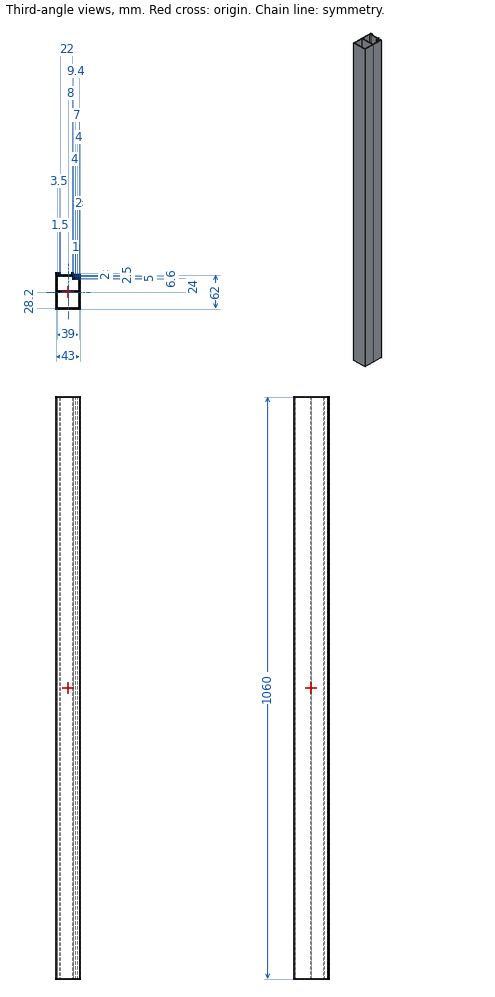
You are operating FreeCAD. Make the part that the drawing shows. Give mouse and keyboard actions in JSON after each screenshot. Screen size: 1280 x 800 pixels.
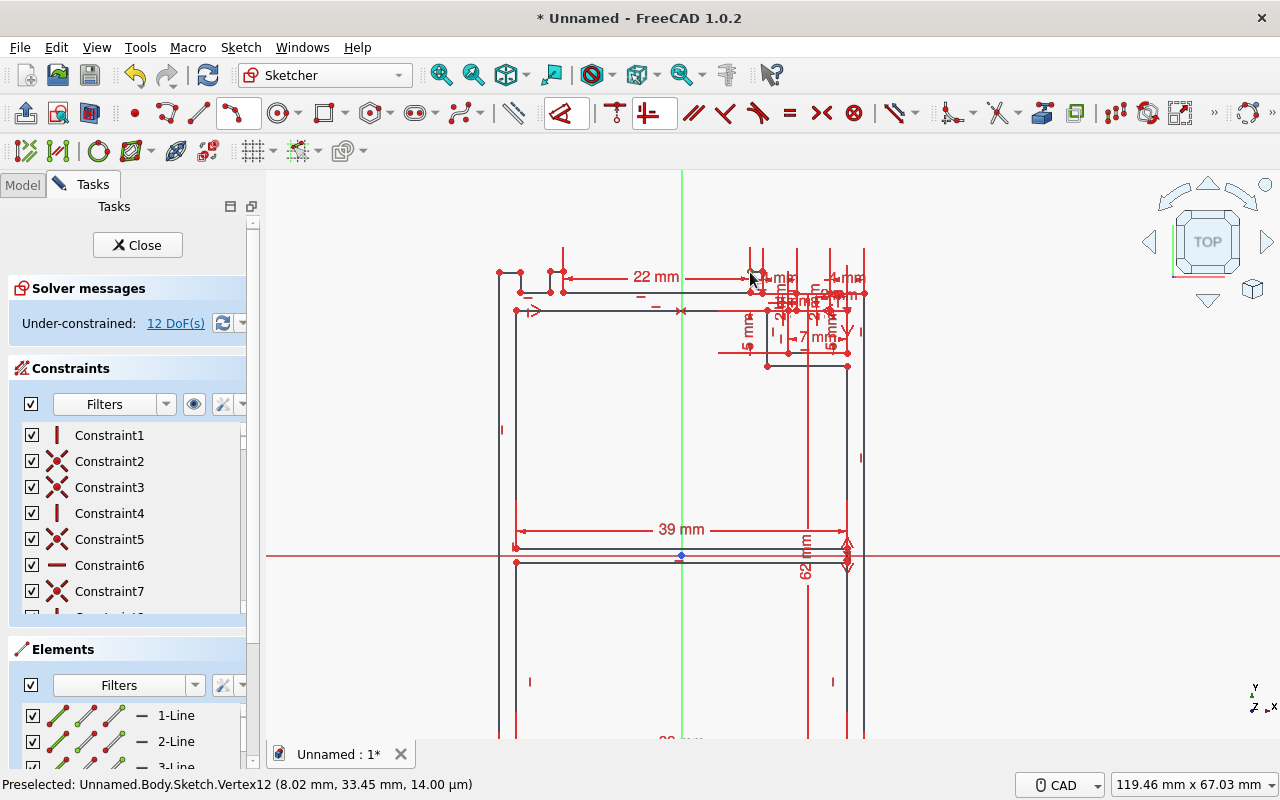
{"action": "key", "text": "l"}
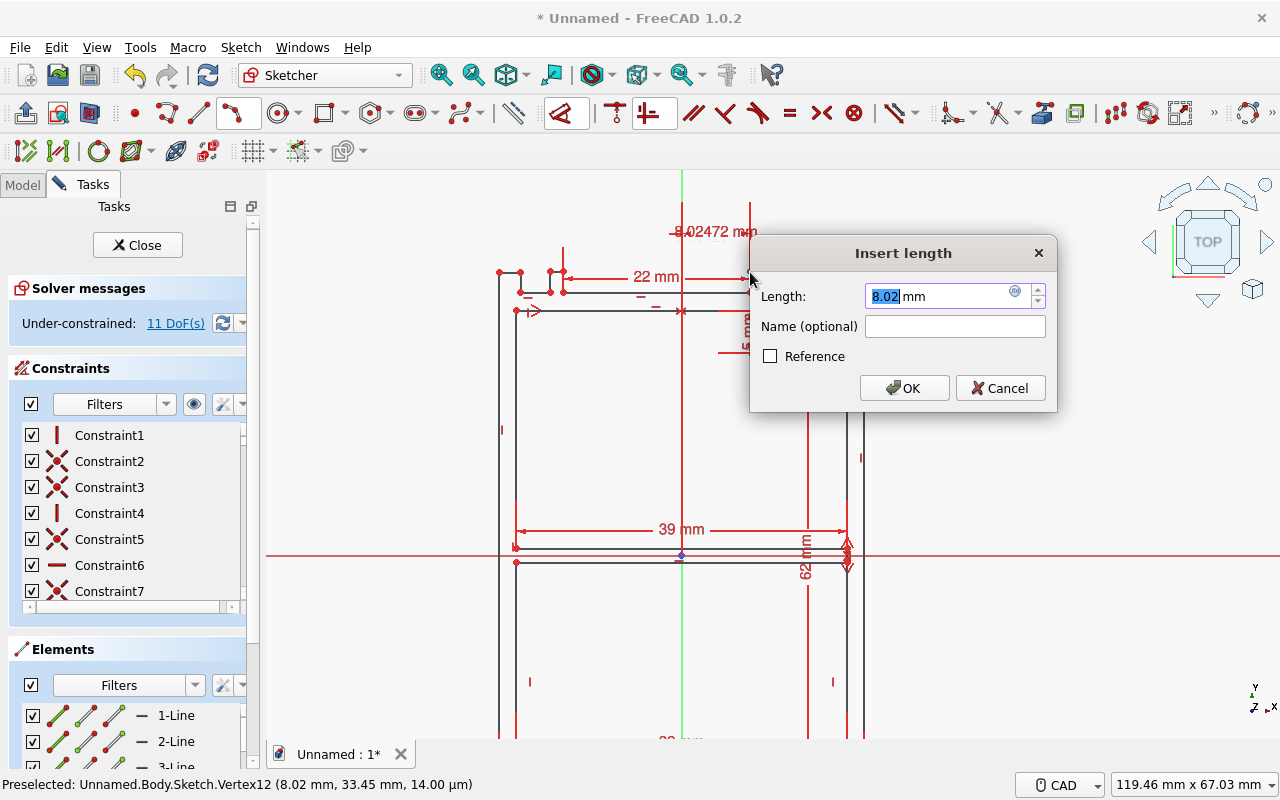
{"action": "type", "text": "8"}
{"action": "key", "text": "Return"}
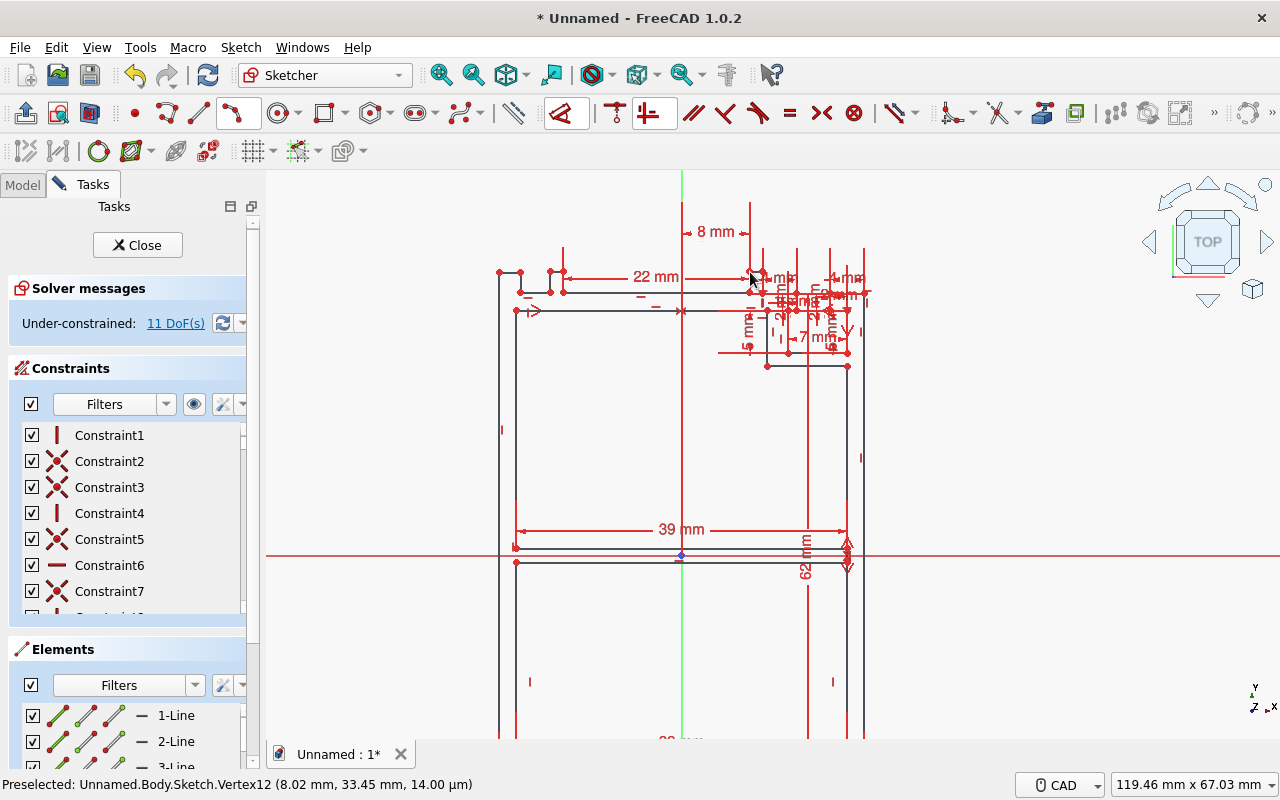
{"action": "scroll", "coordinate": [763, 283], "scroll_direction": "up", "scroll_amount": 4}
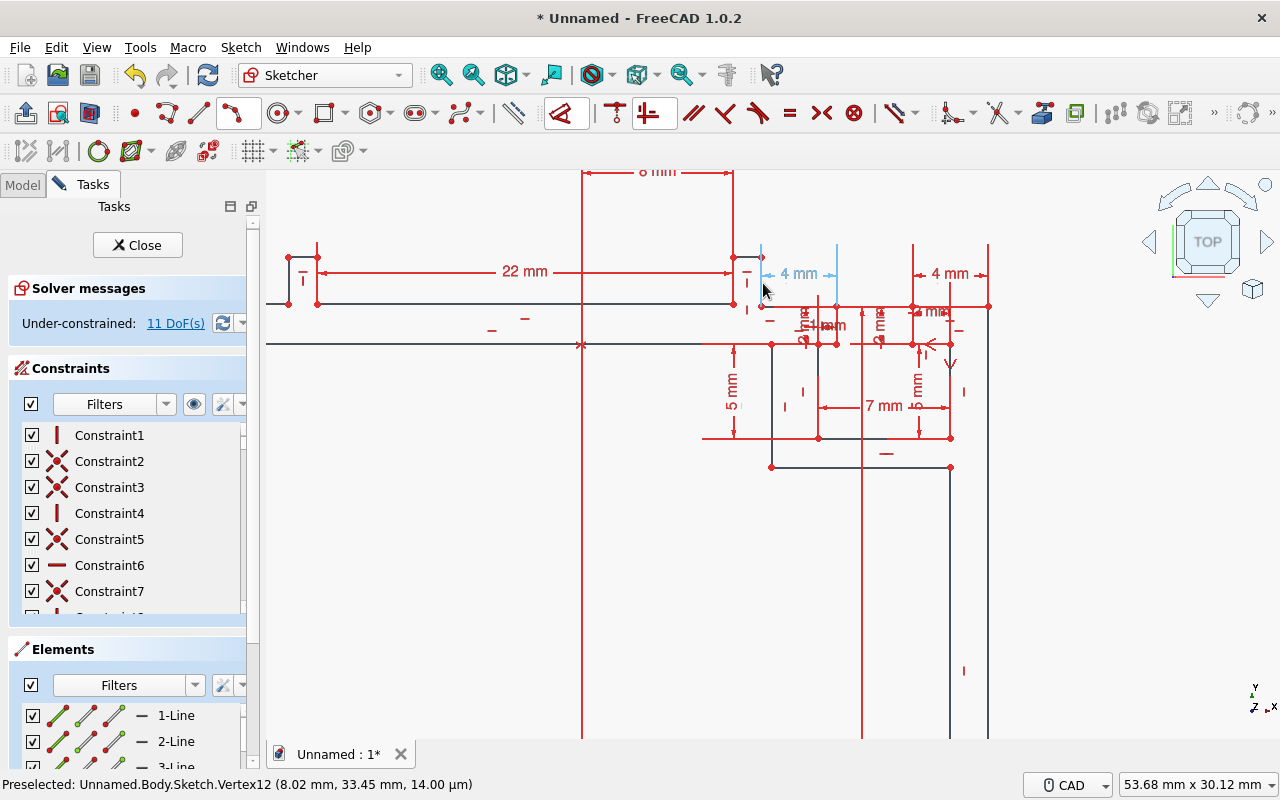
{"action": "left_click", "coordinate": [761, 282]}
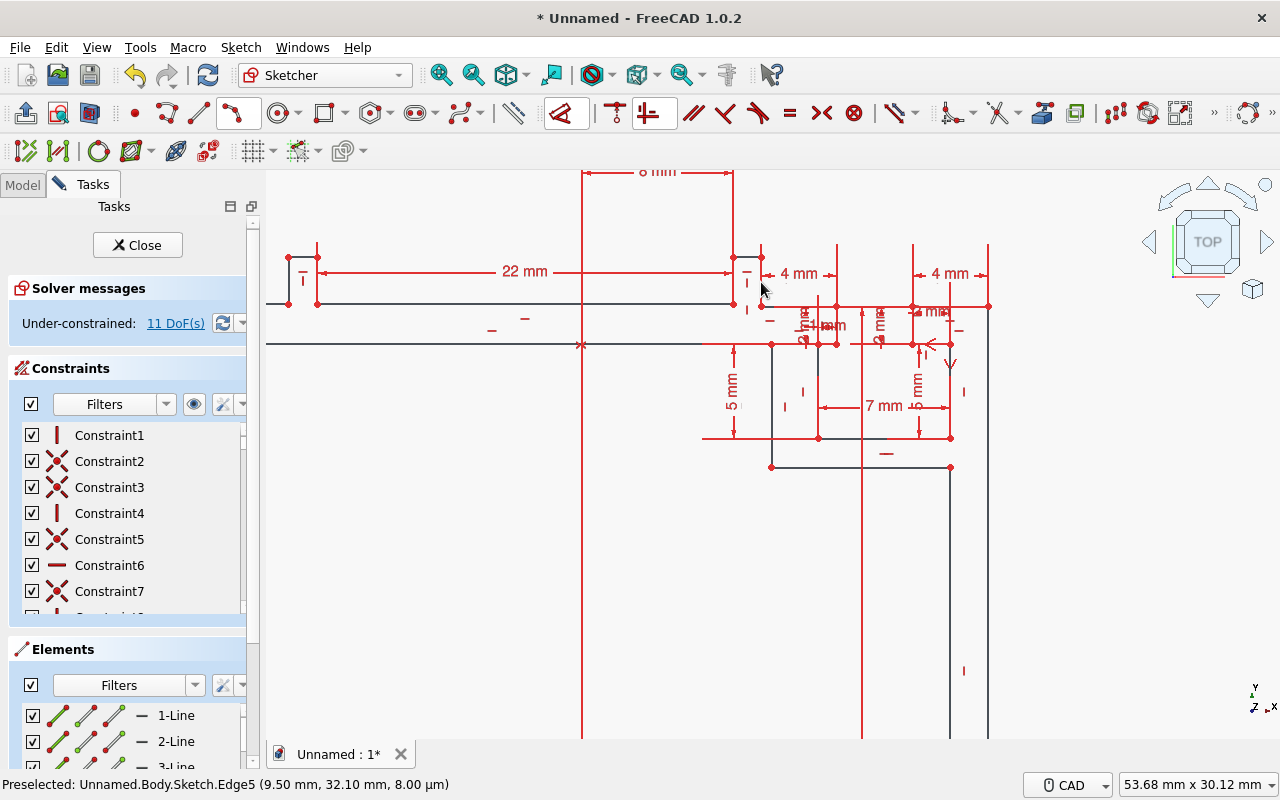
{"action": "key", "text": "i"}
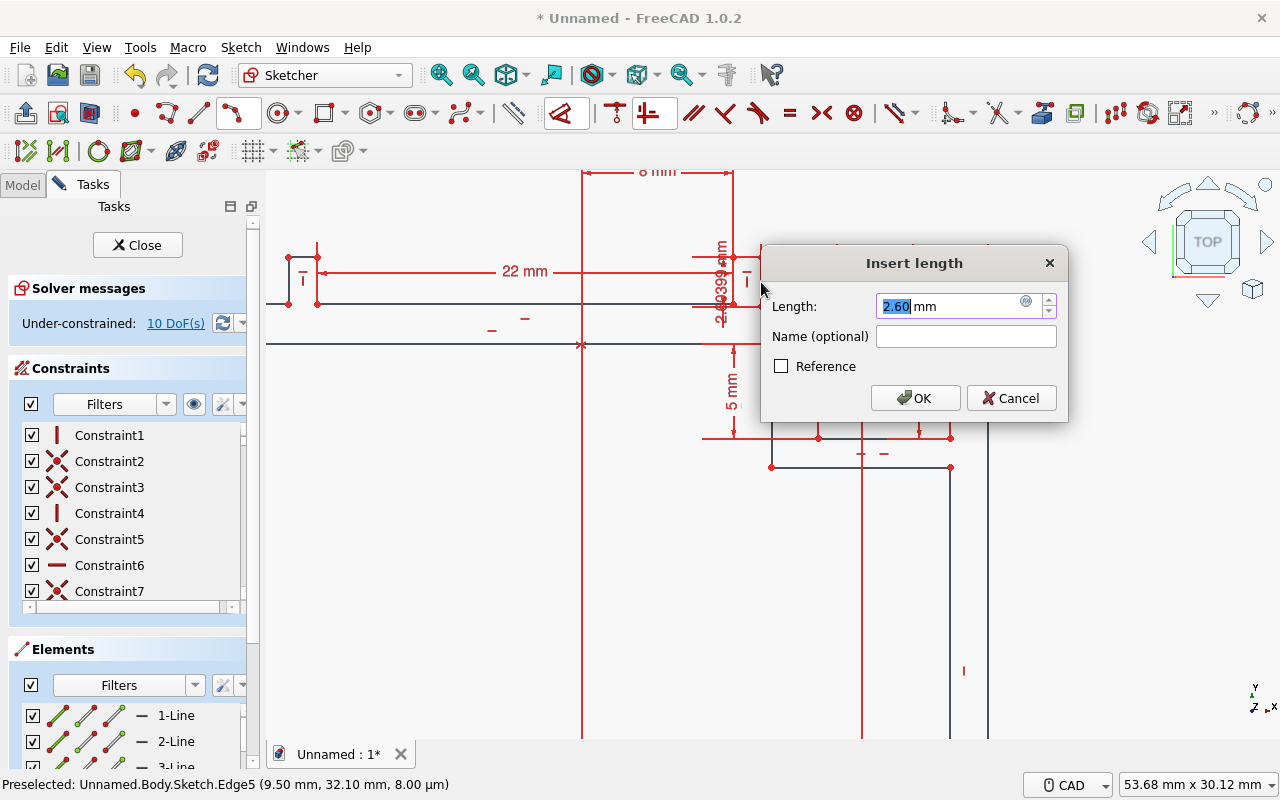
{"action": "type", "text": "2.5"}
{"action": "key", "text": "Return"}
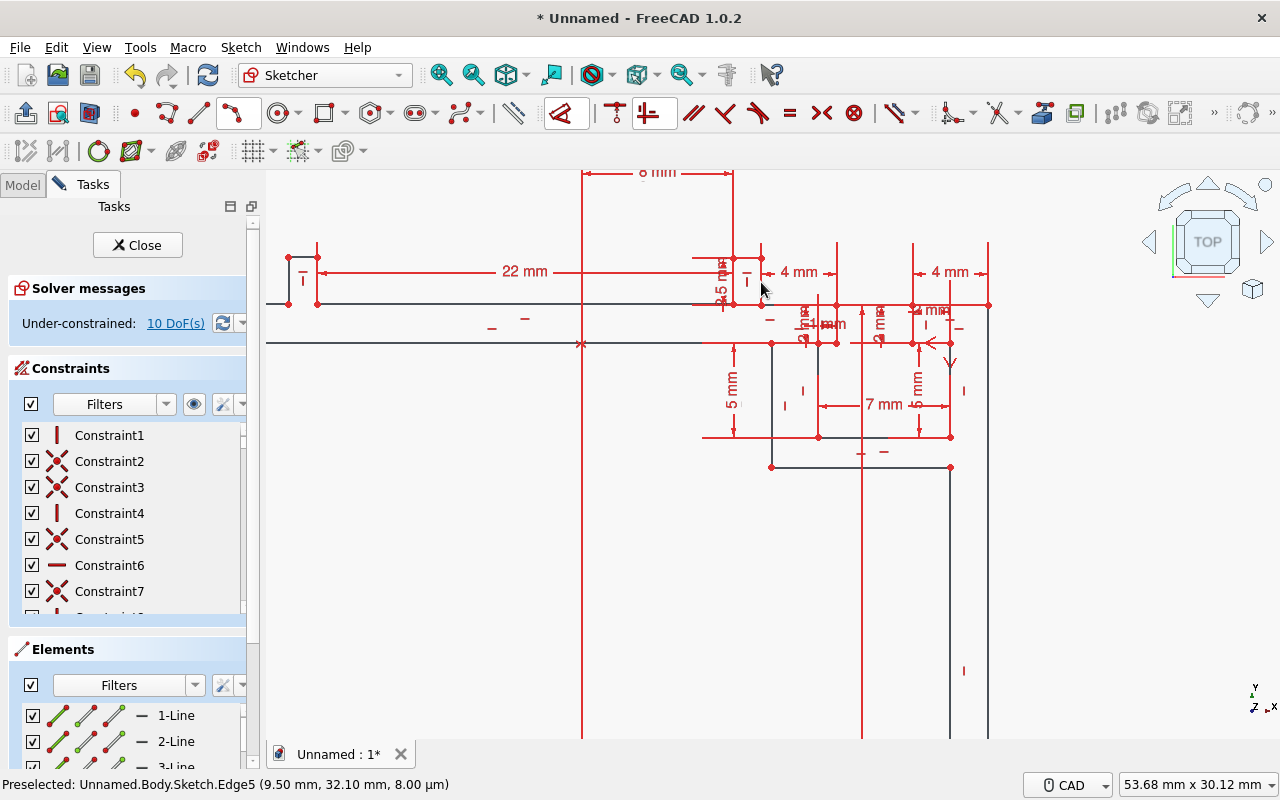
{"action": "left_click", "coordinate": [733, 272]}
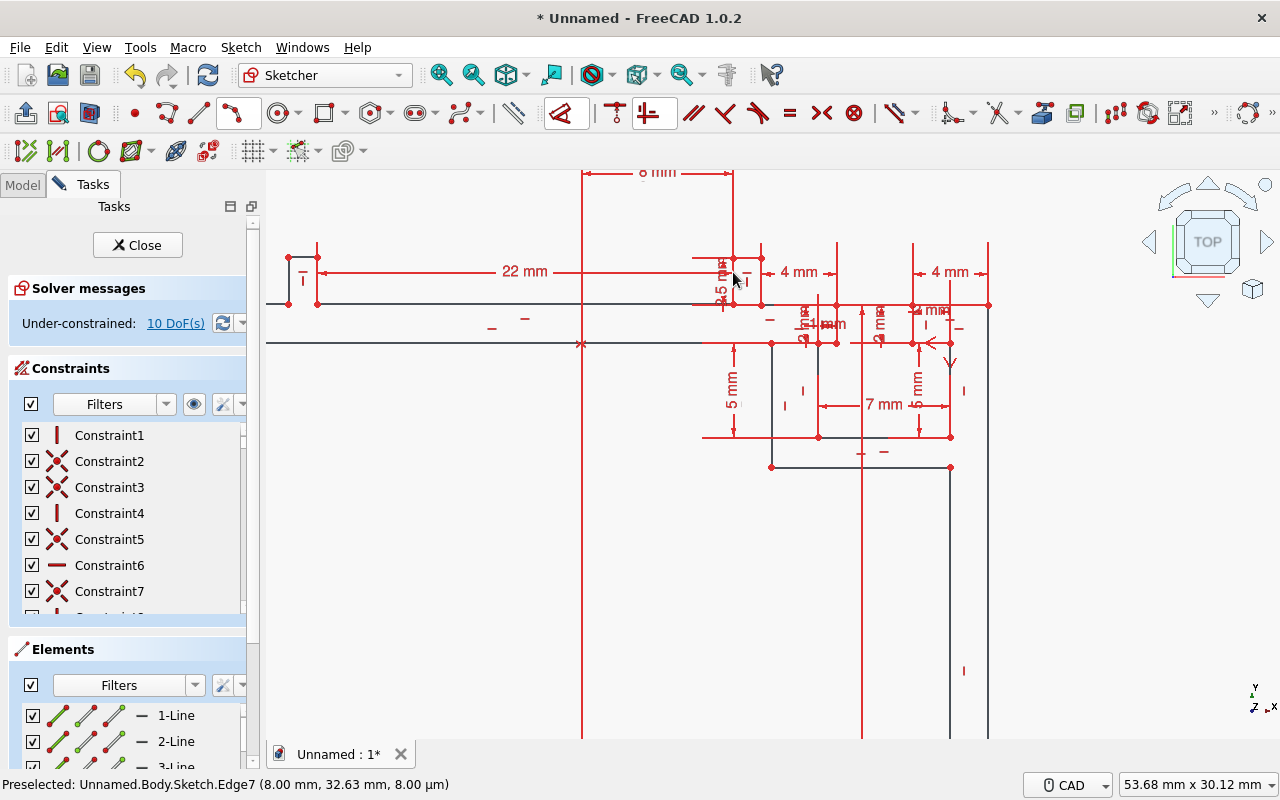
{"action": "key", "text": "i"}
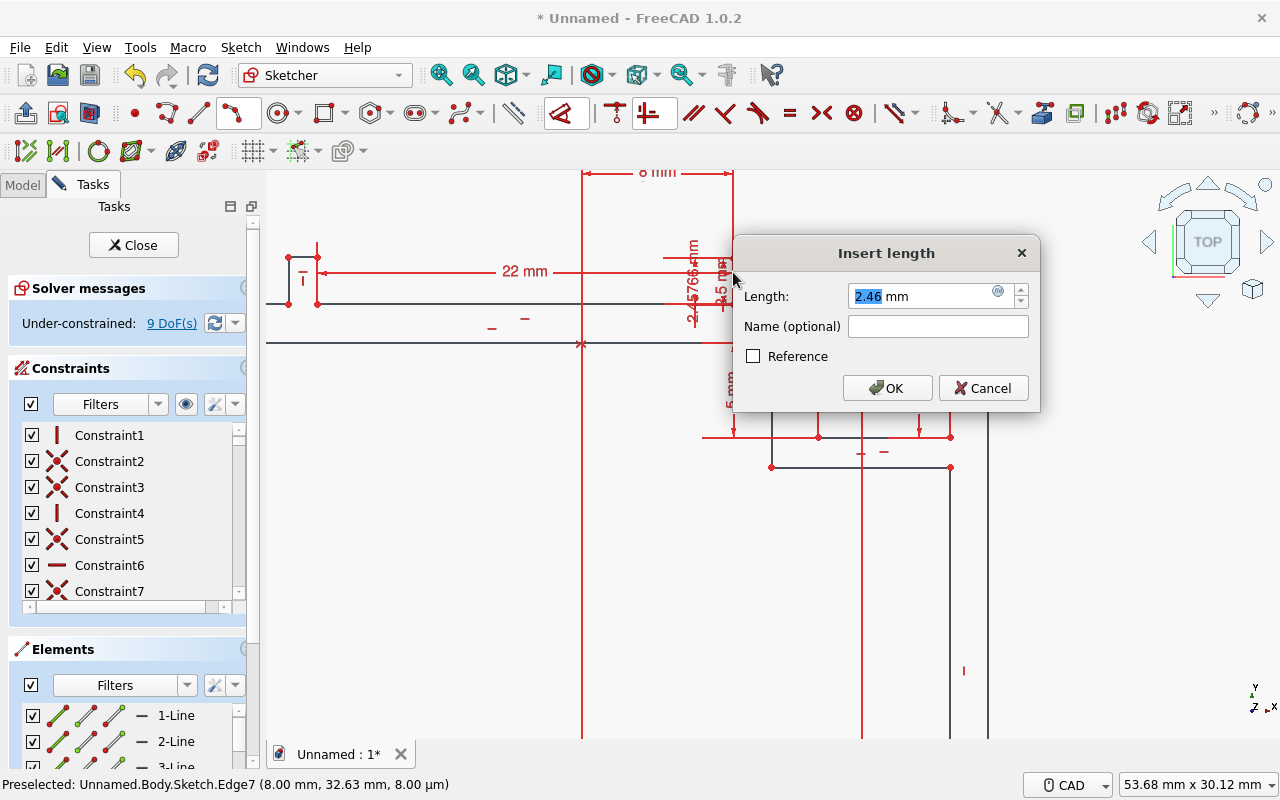
{"action": "type", "text": "2.5"}
{"action": "key", "text": "Return"}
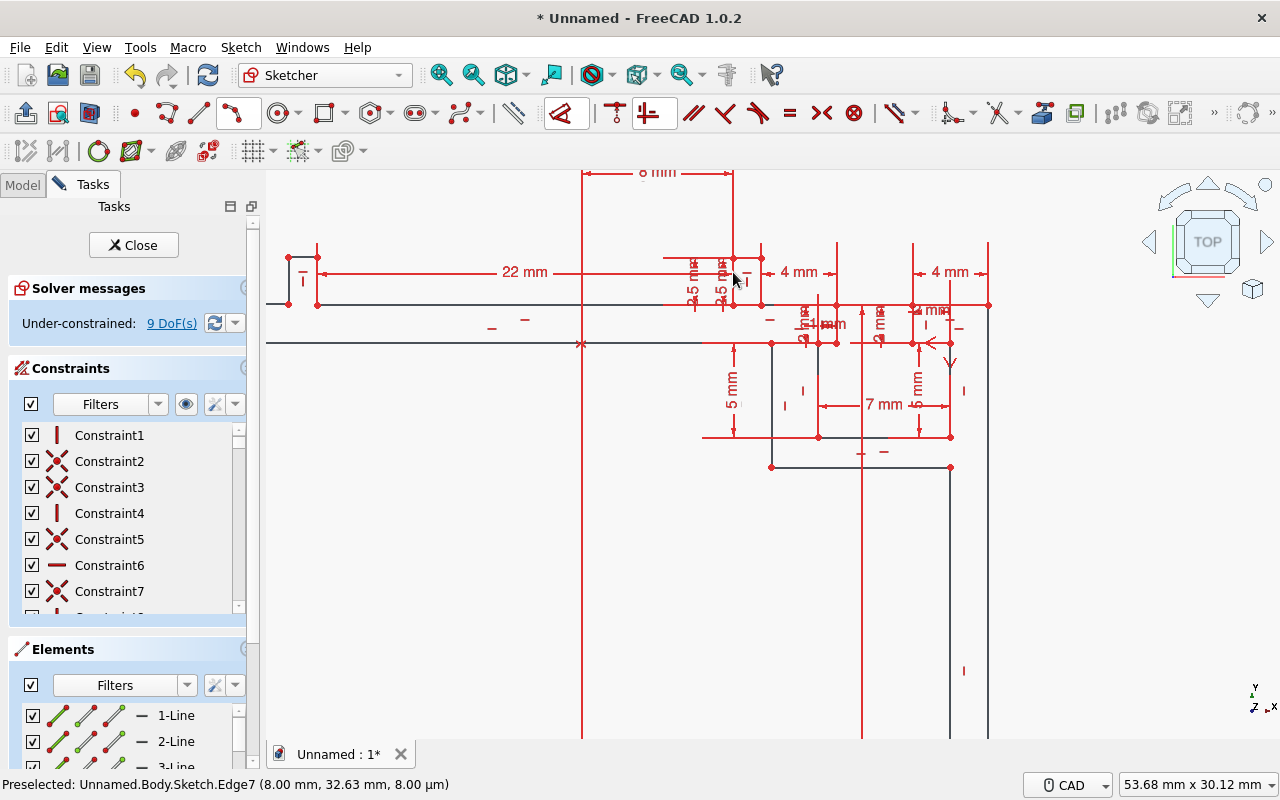
{"action": "left_click", "coordinate": [317, 291]}